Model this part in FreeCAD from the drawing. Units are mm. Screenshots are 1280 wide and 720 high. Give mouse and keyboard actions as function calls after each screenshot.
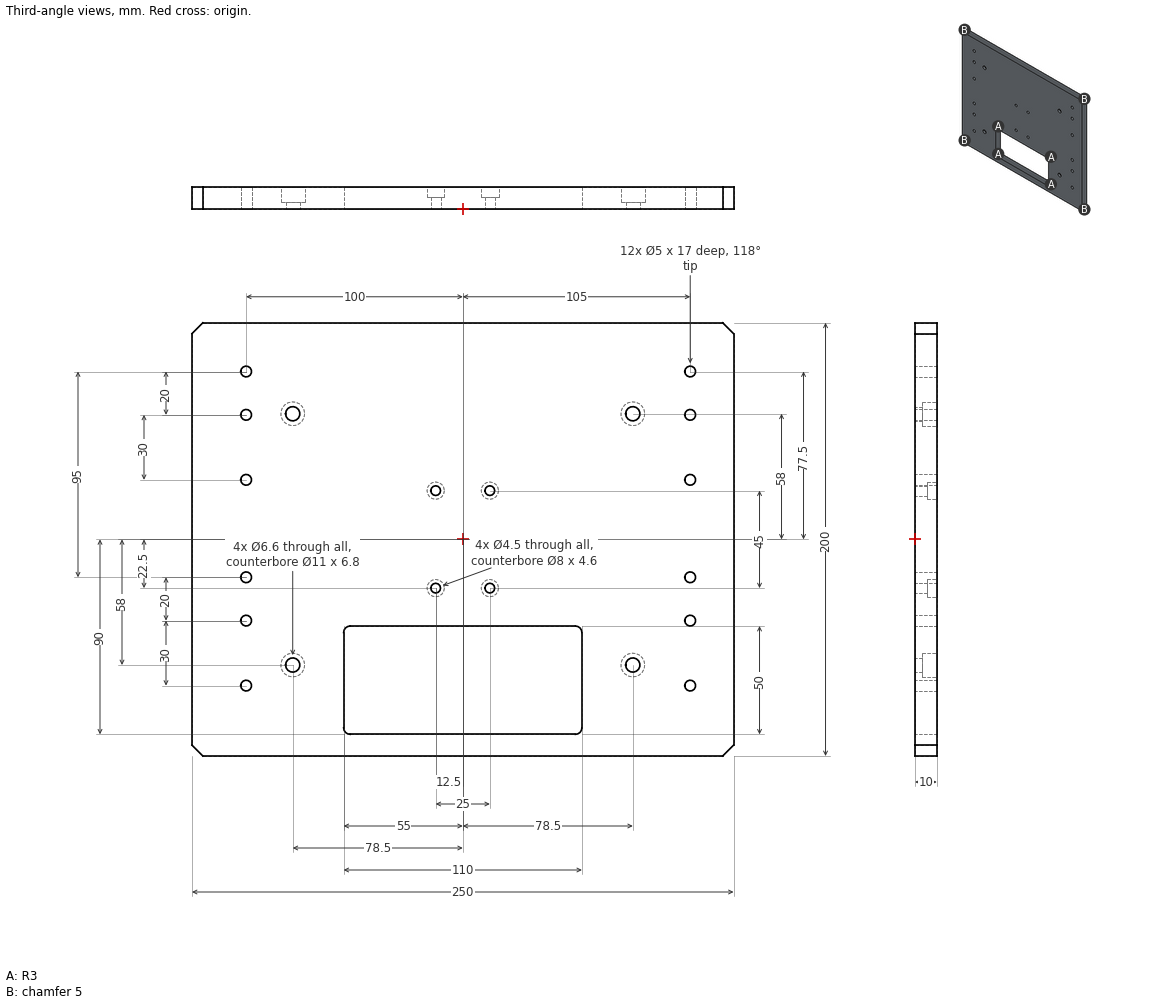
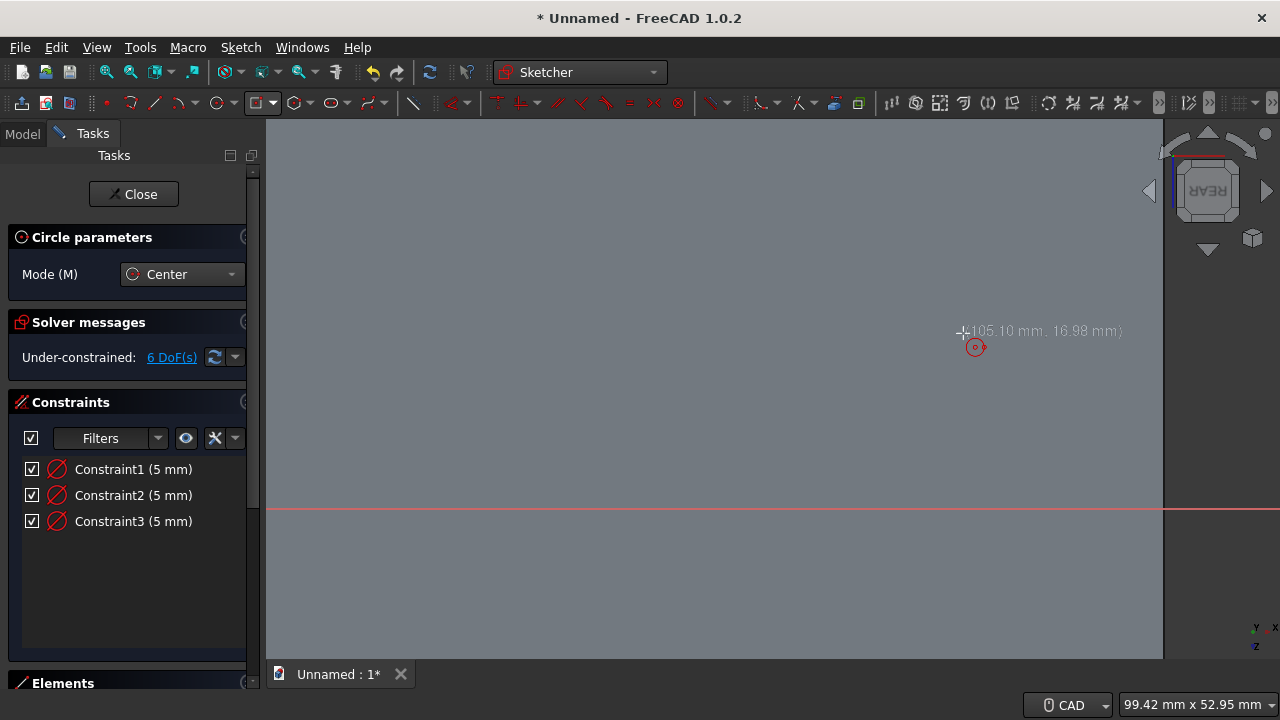
scroll(963, 333, down, 7)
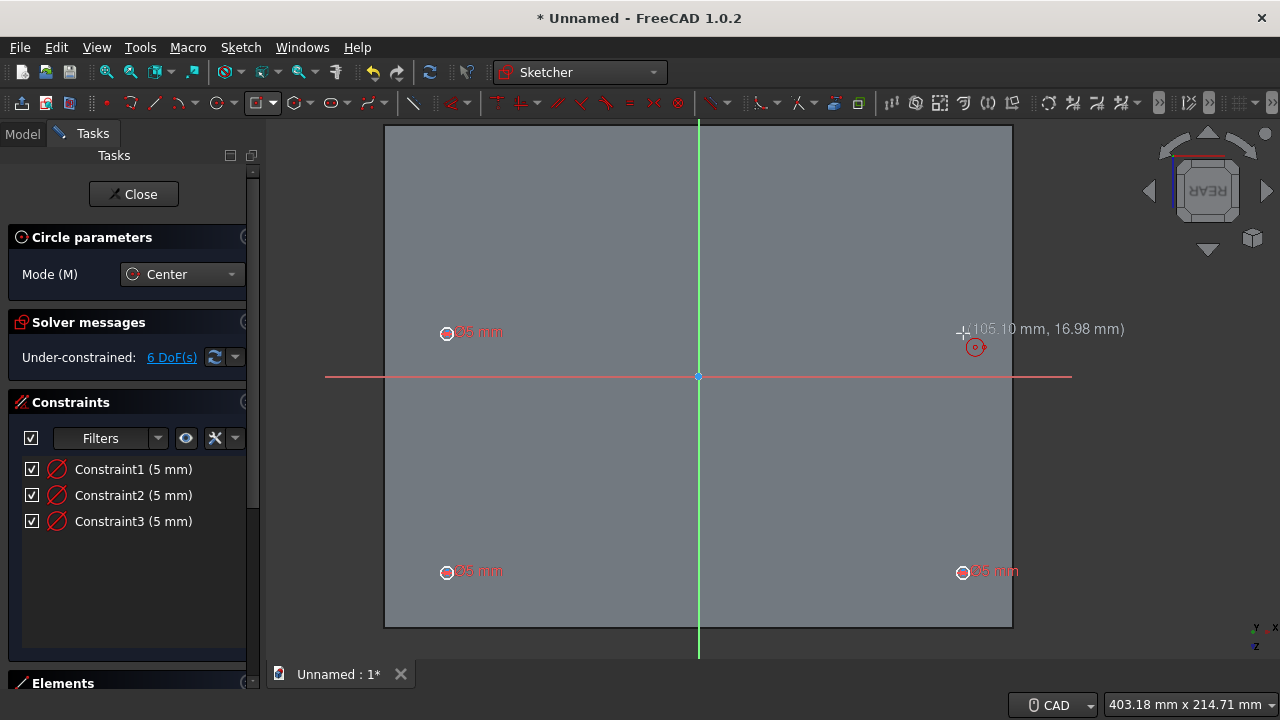
click(963, 333)
move(967, 328)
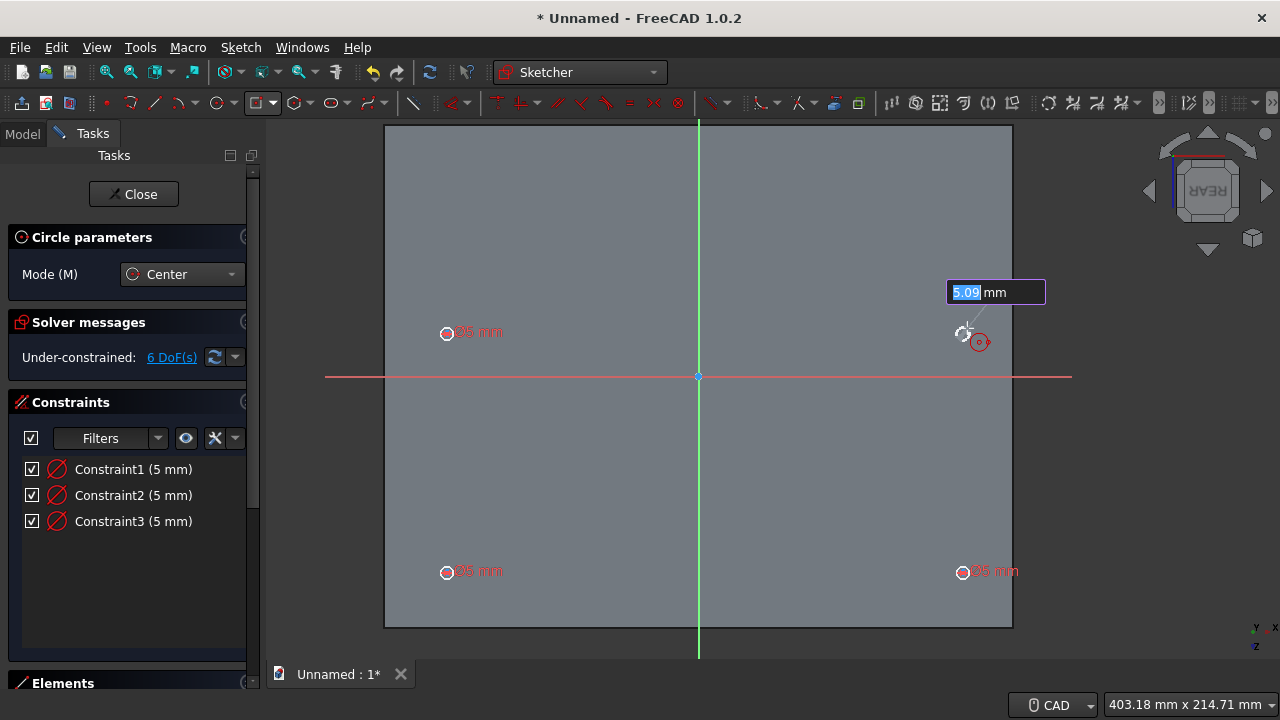
text(5)
key(Return)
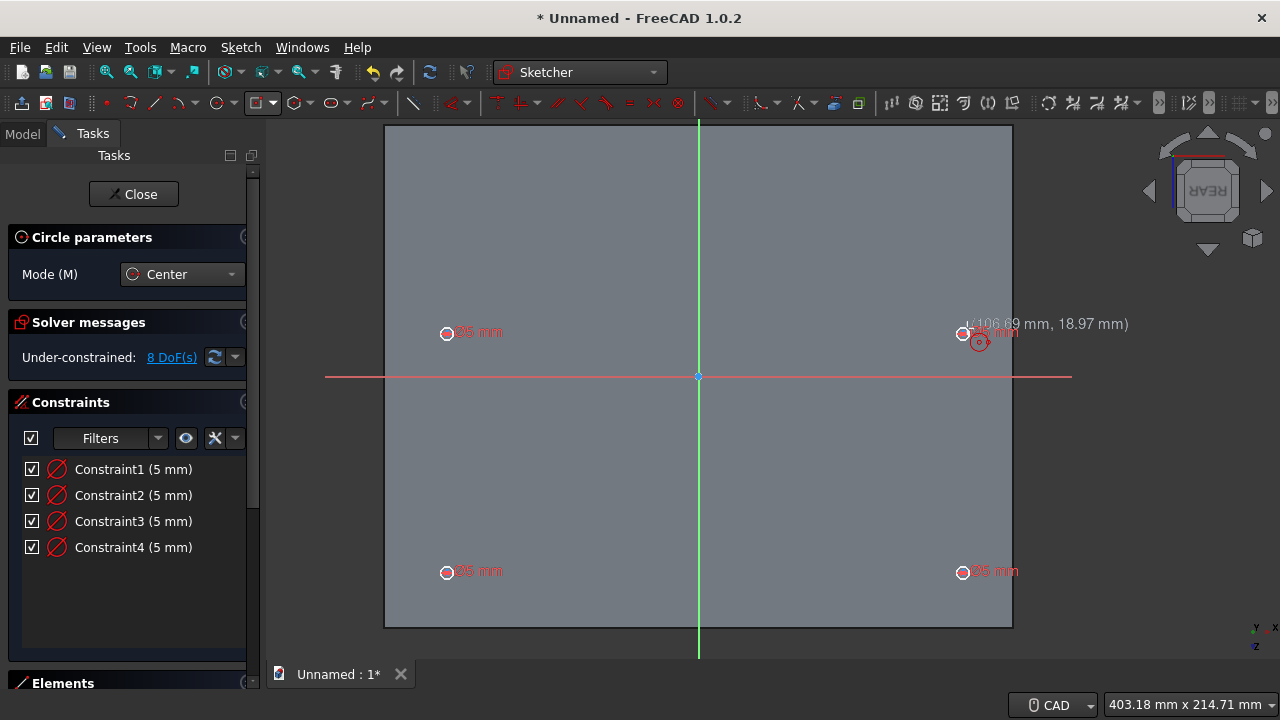
scroll(447, 282, up, 7)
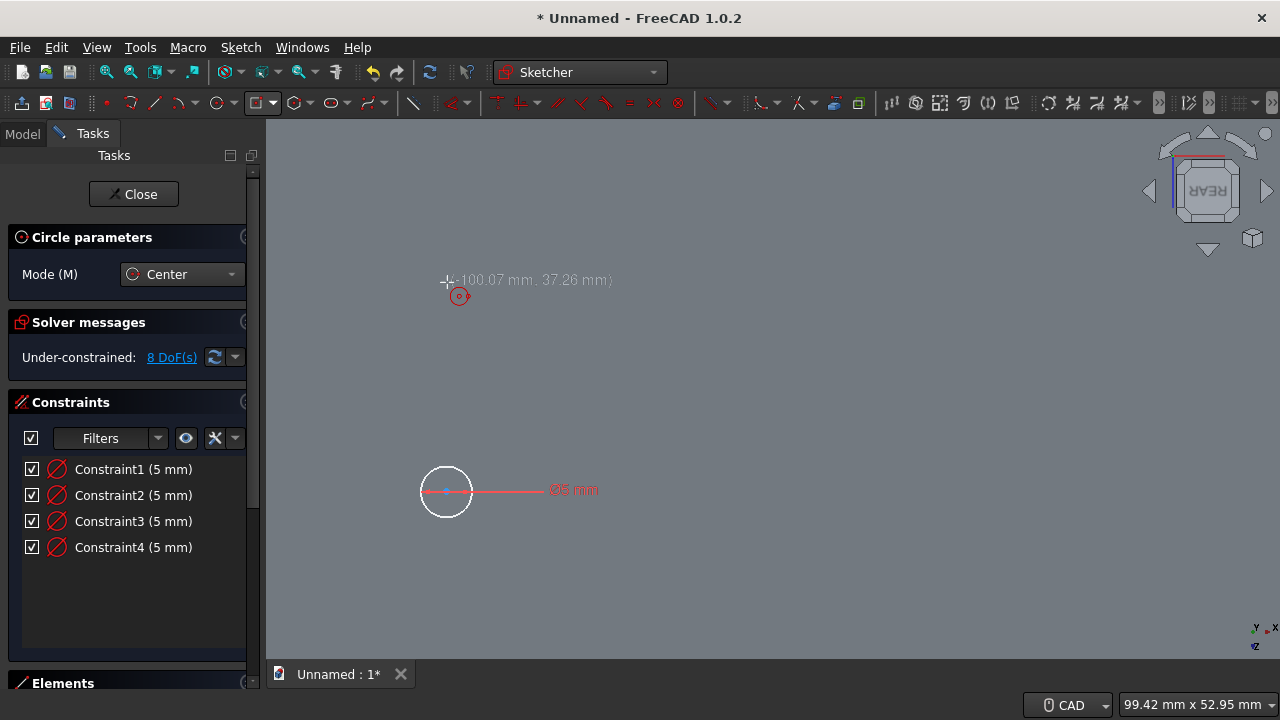
scroll(447, 282, down, 7)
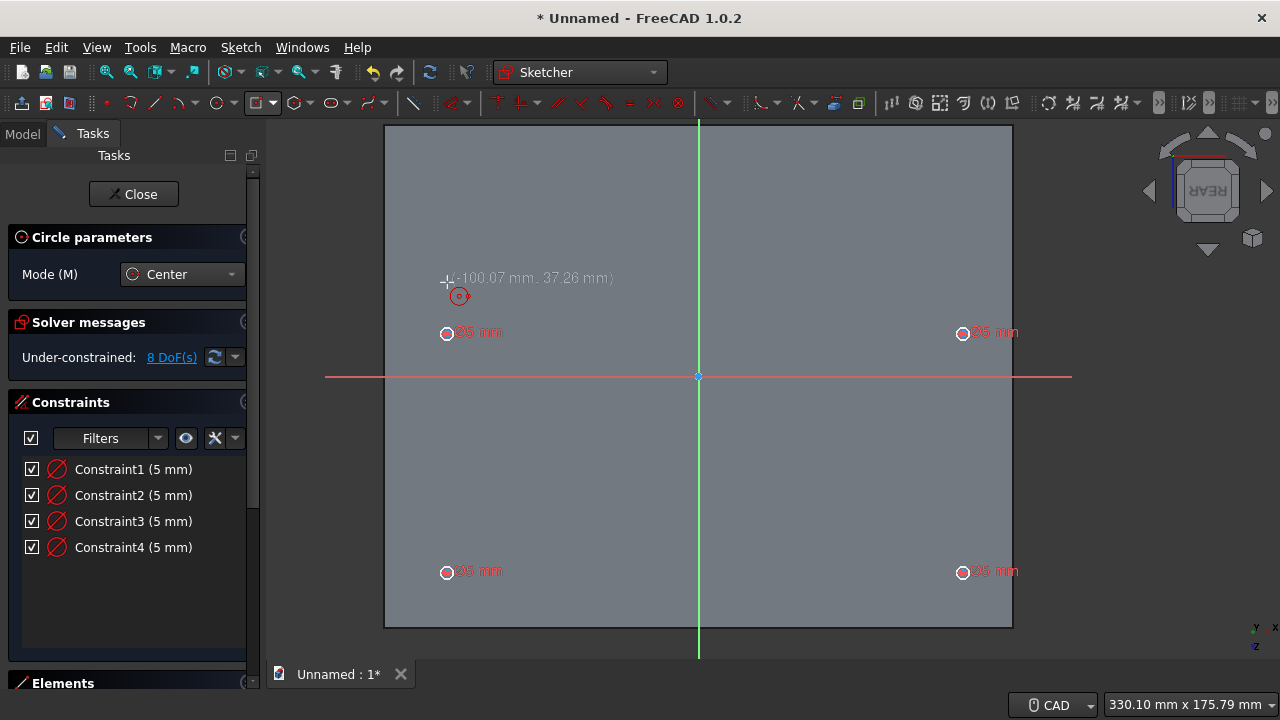
click(447, 282)
move(452, 278)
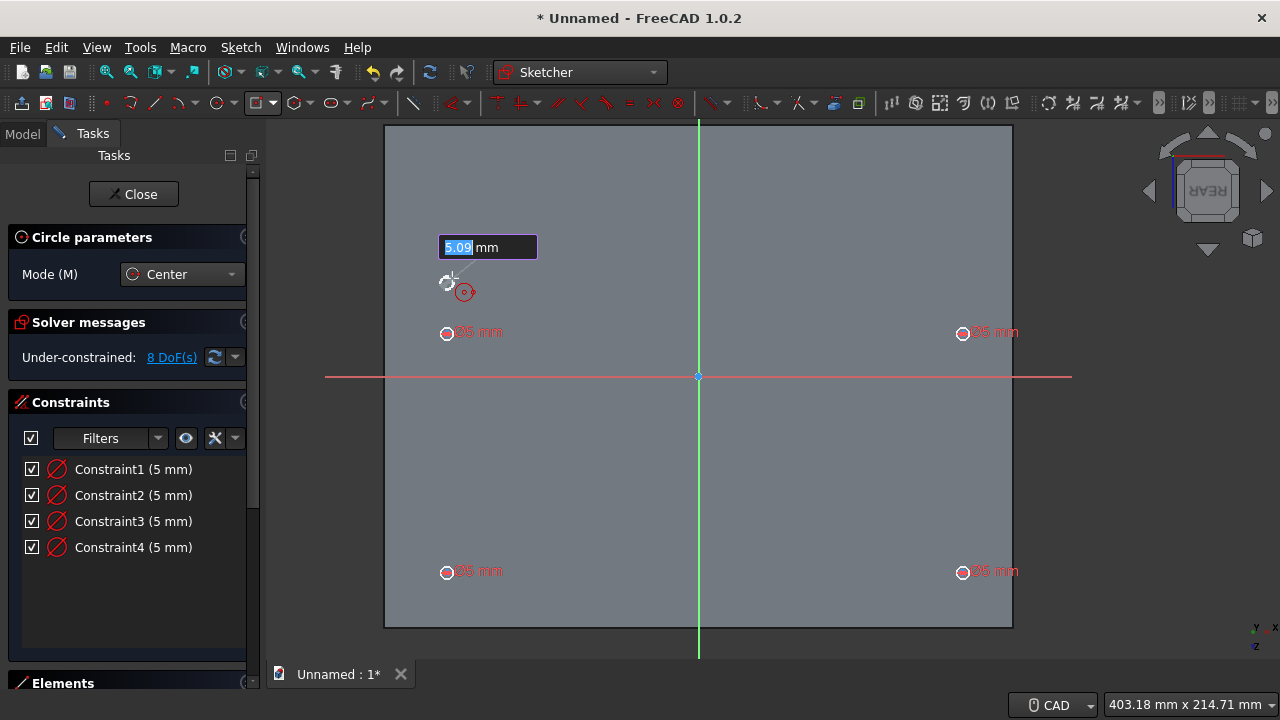
text(5)
key(Return)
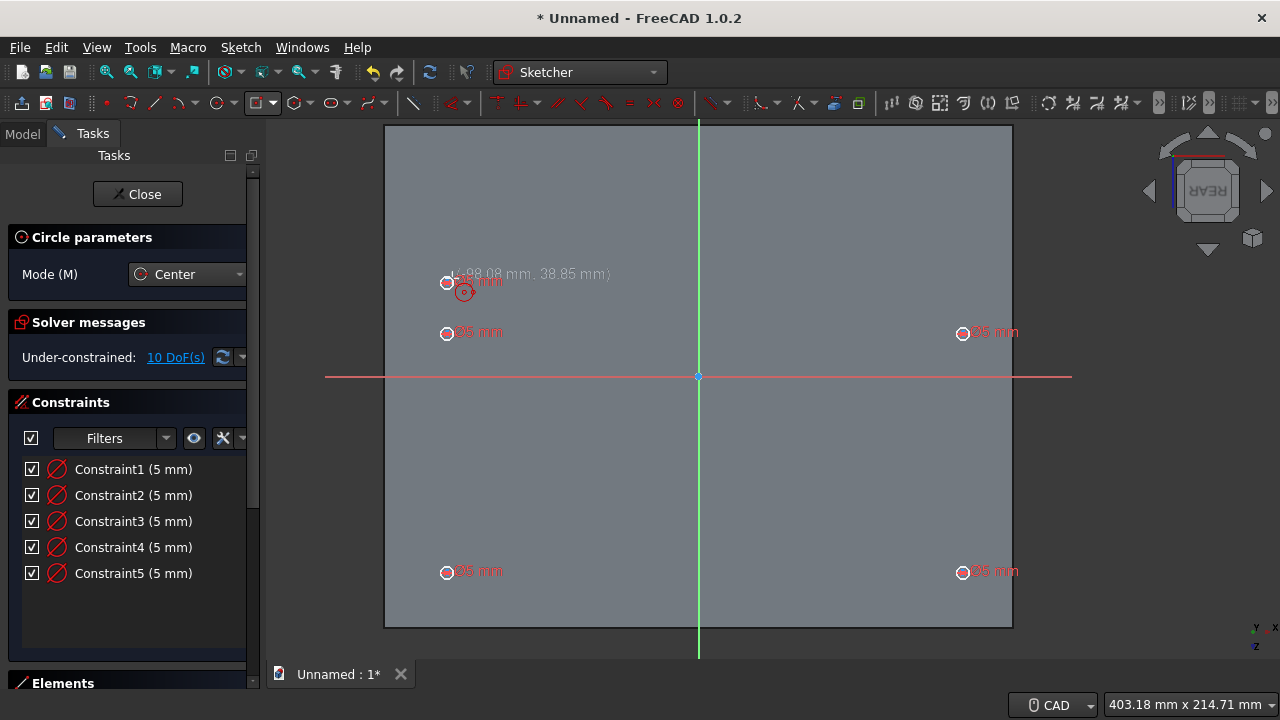
scroll(447, 207, up, 7)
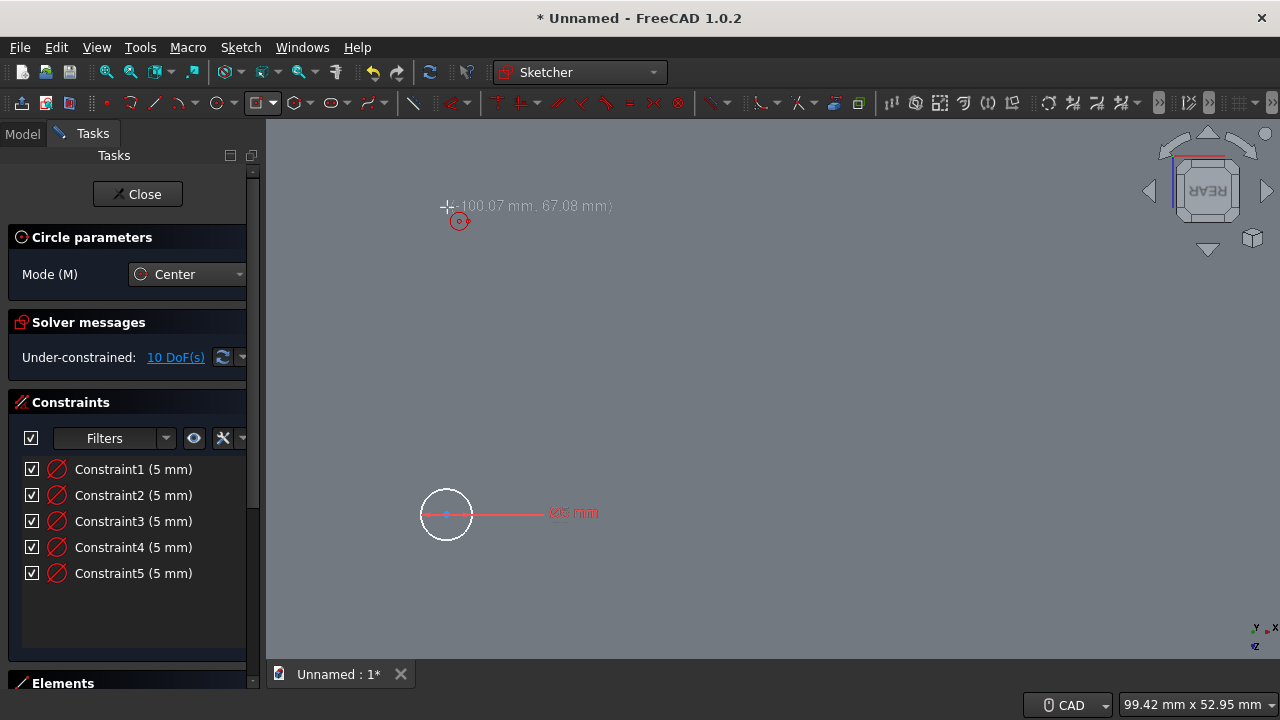
scroll(447, 207, down, 7)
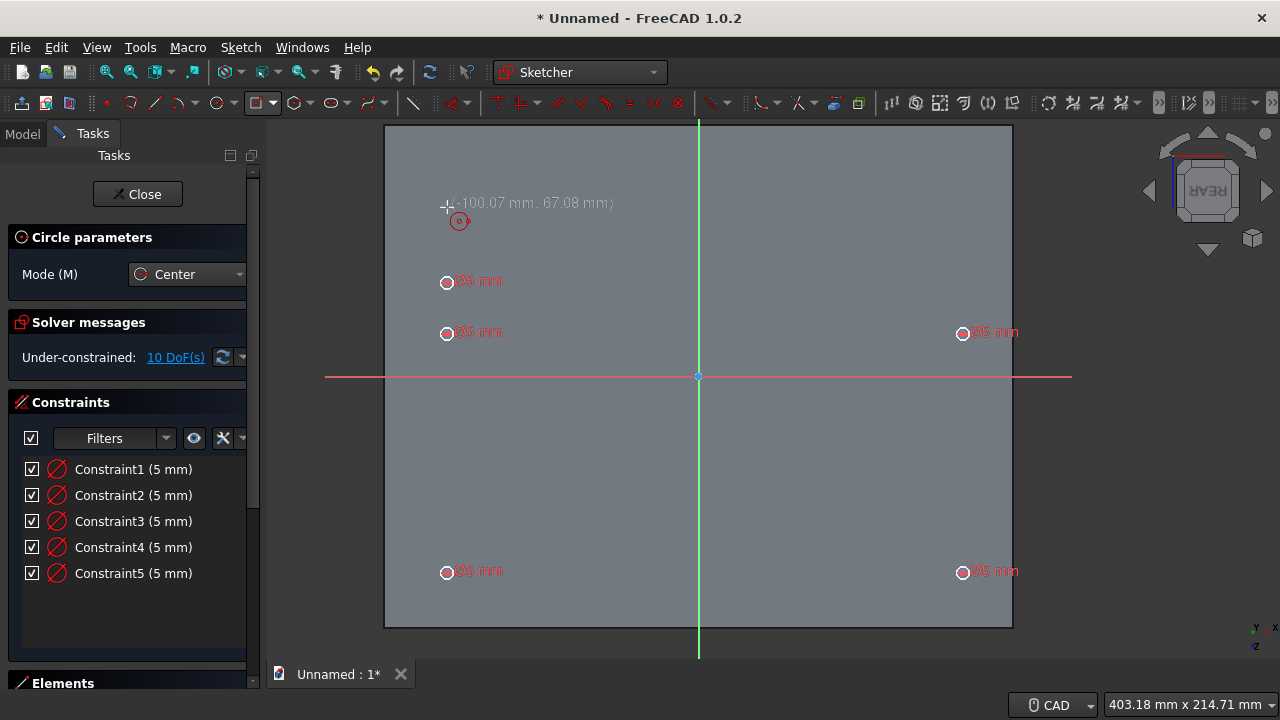
click(447, 207)
move(452, 202)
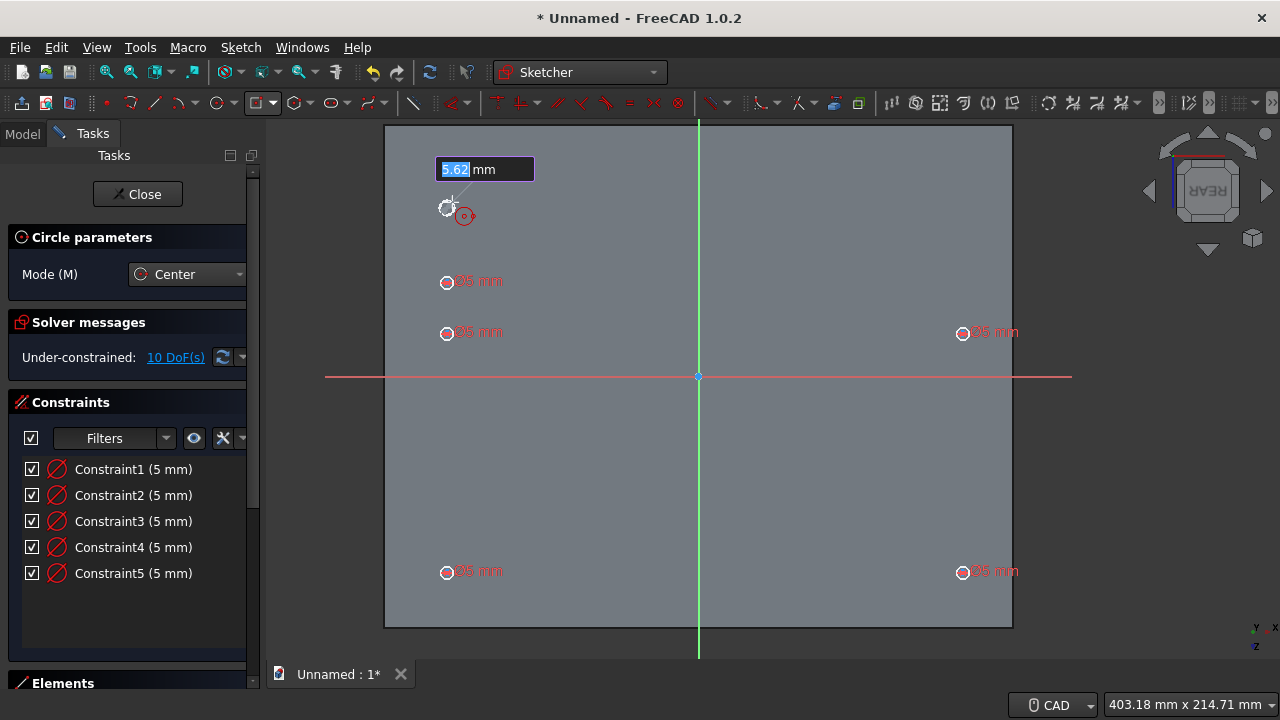
text(5)
key(Return)